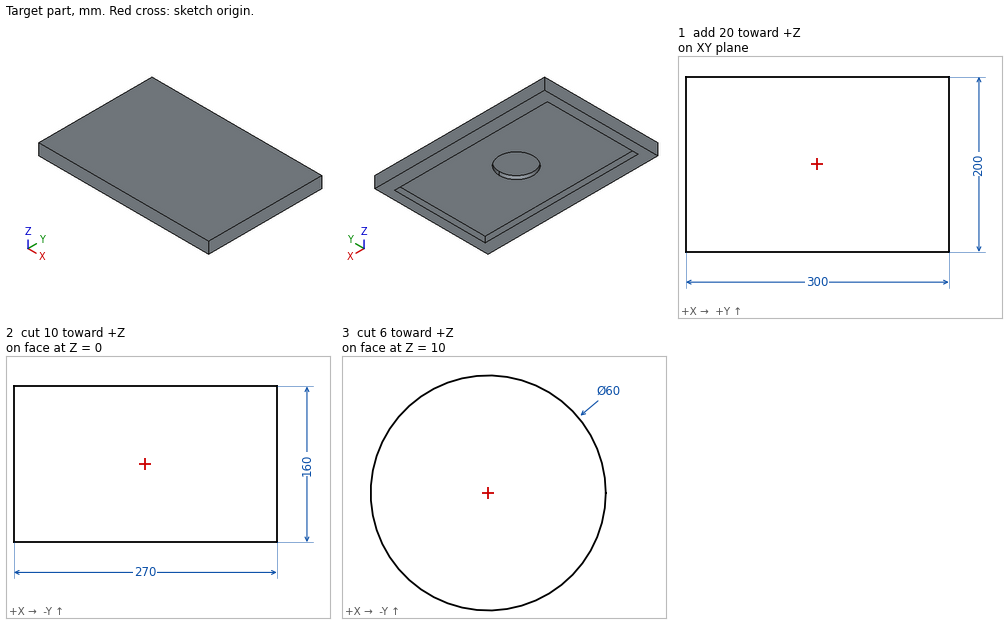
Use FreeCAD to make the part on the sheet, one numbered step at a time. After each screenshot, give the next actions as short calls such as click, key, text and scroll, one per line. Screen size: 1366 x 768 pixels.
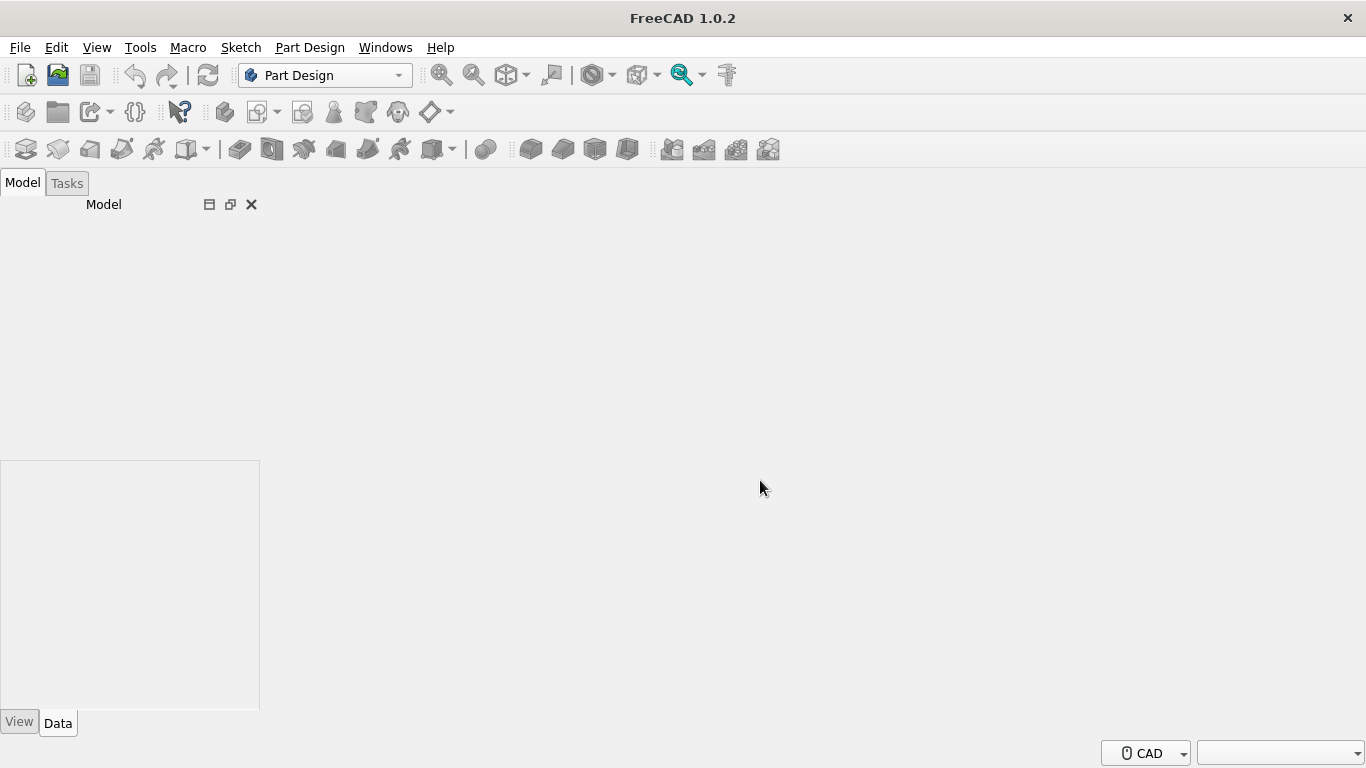
key(ctrl+n)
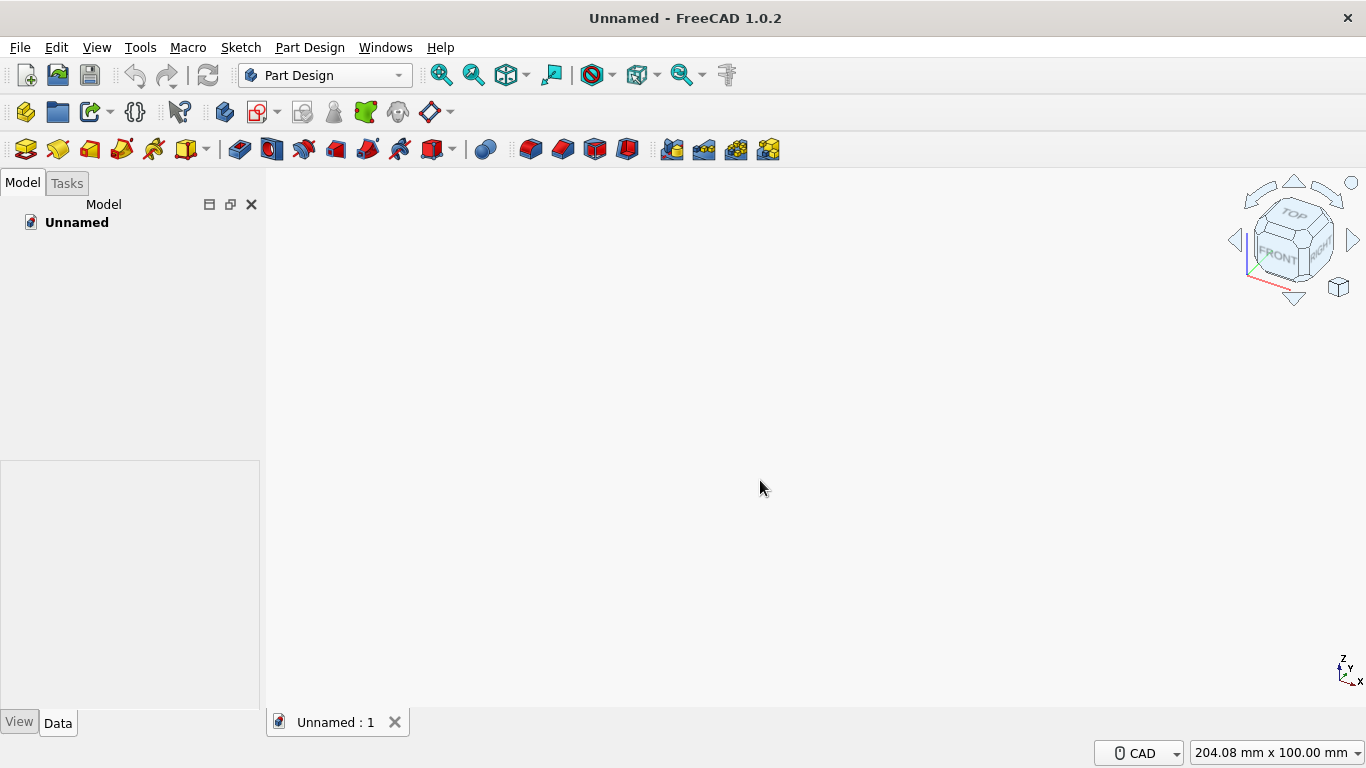
click(258, 112)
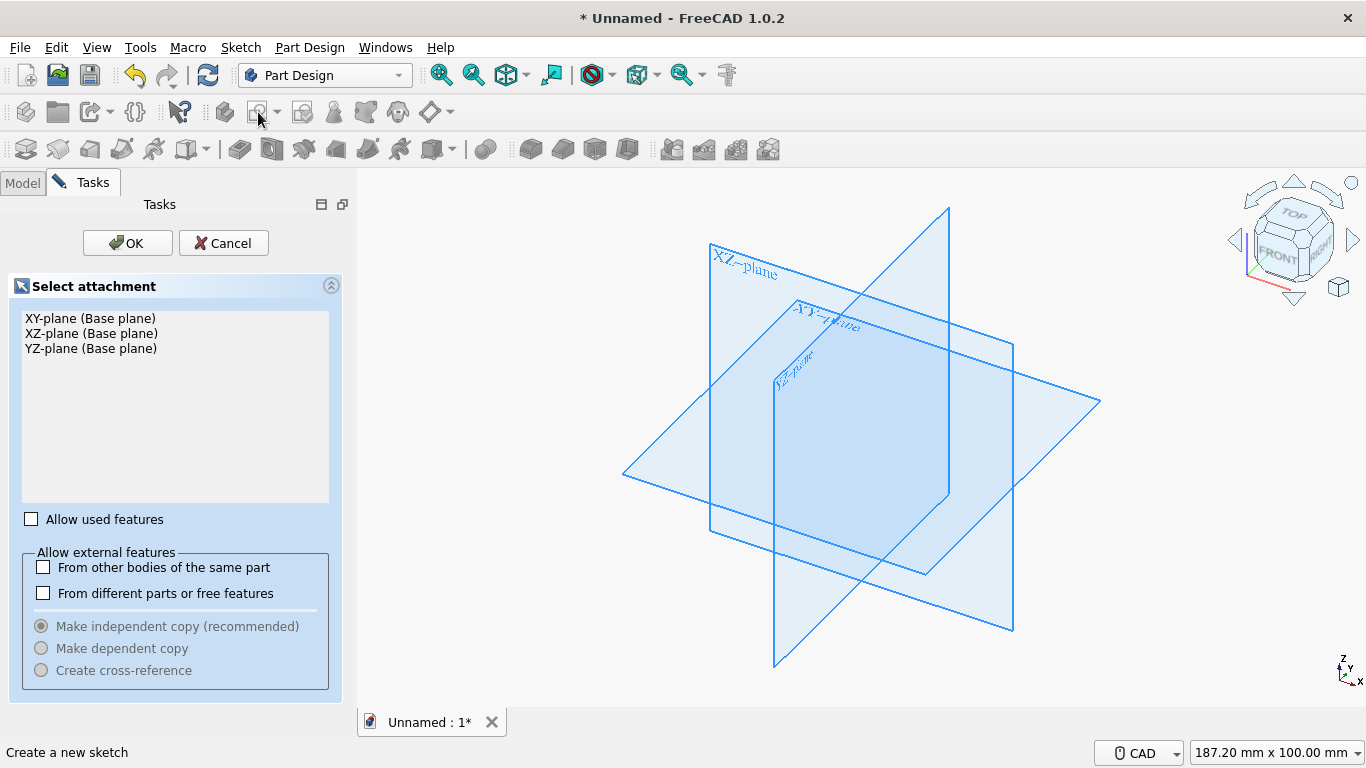
click(82, 318)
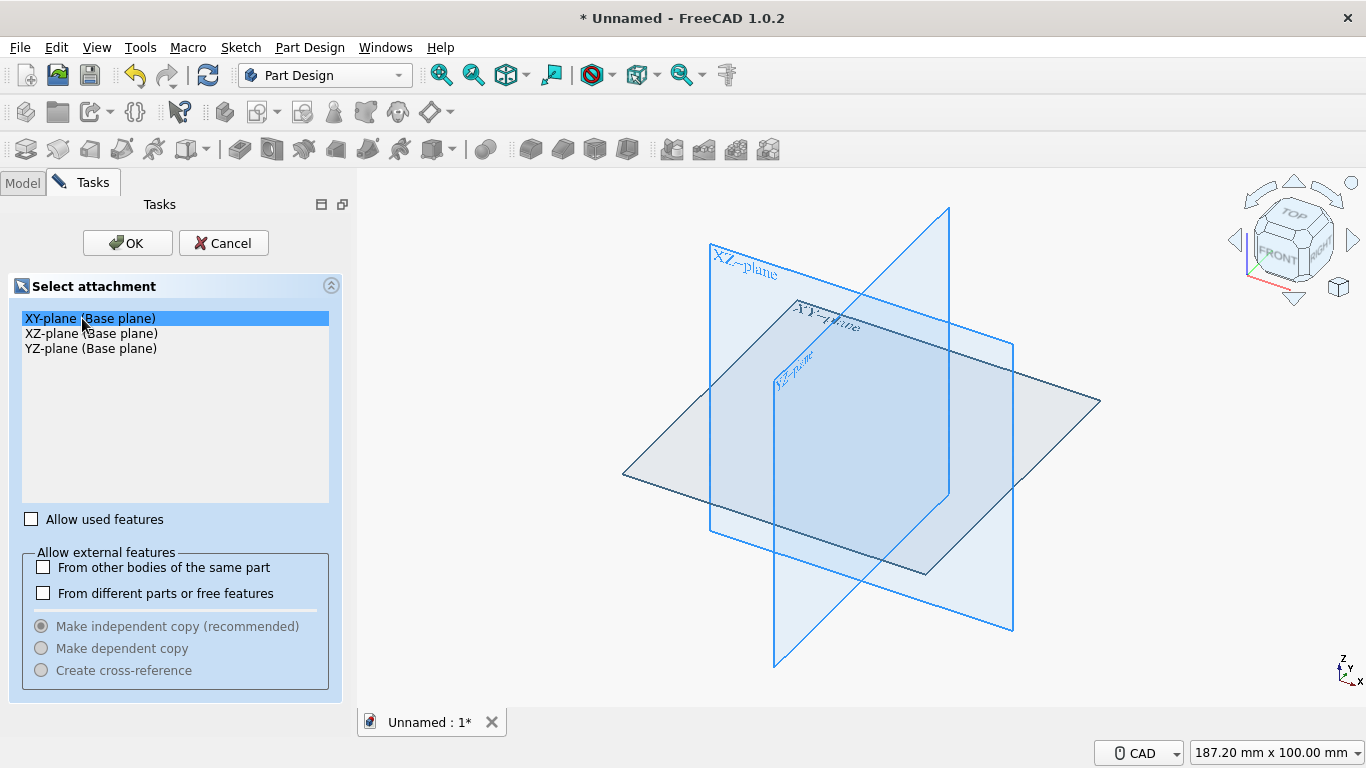
click(128, 243)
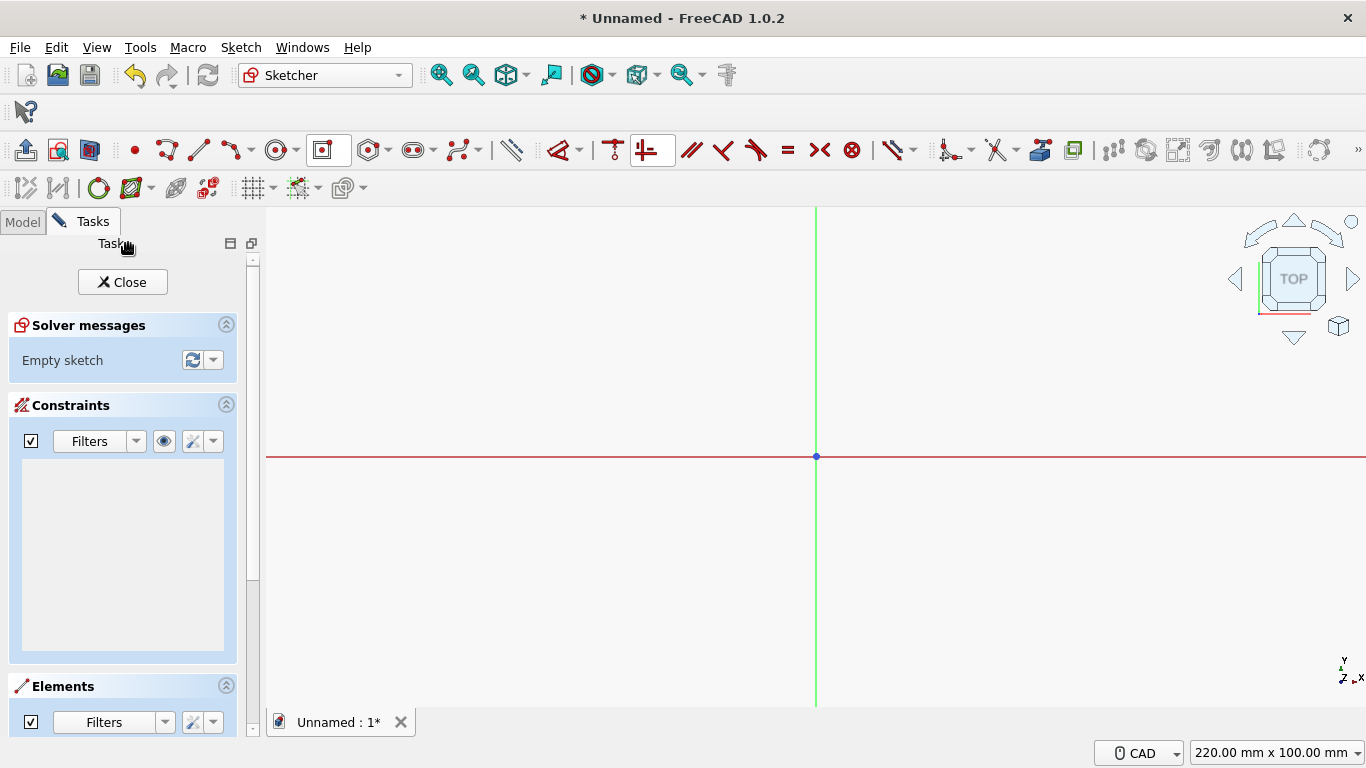
scroll(718, 457, down, 6)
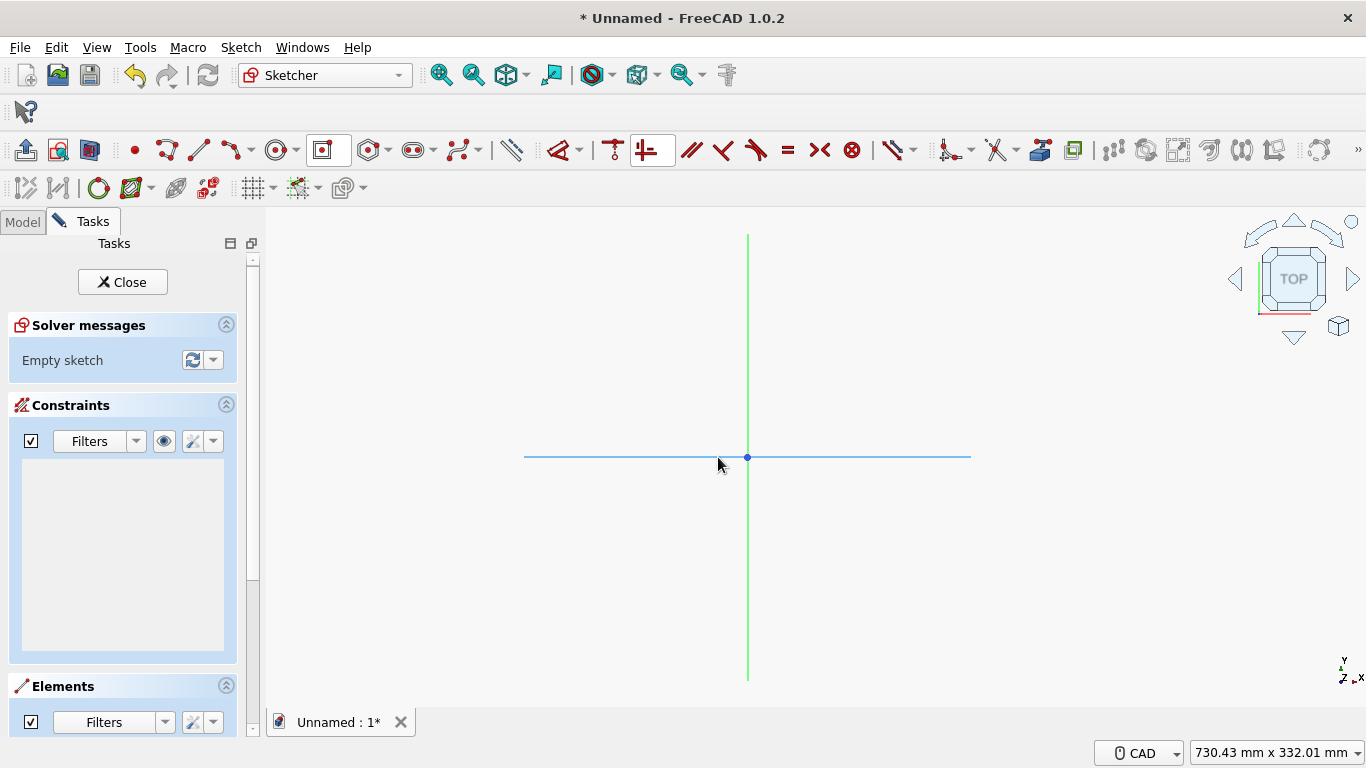
key(g)
key(v)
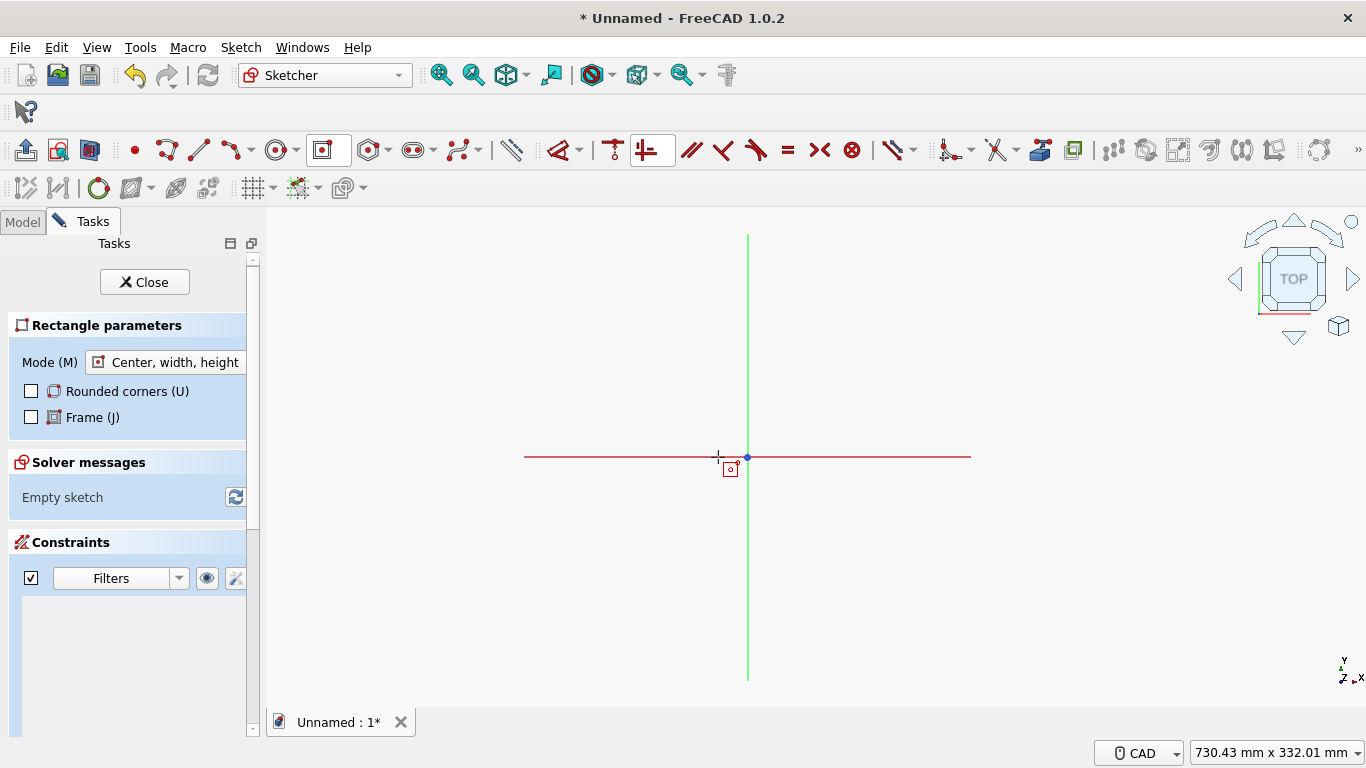
click(748, 457)
click(974, 307)
key(Escape)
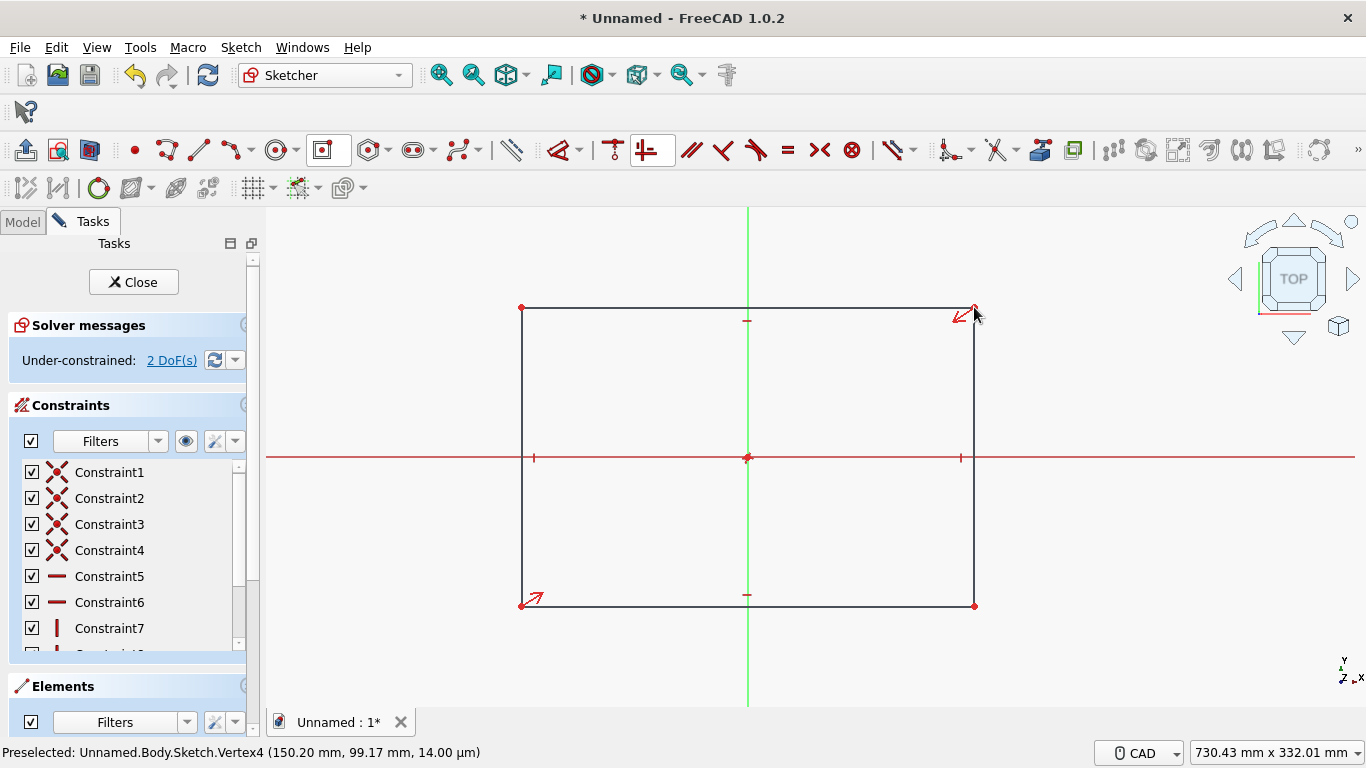
click(657, 607)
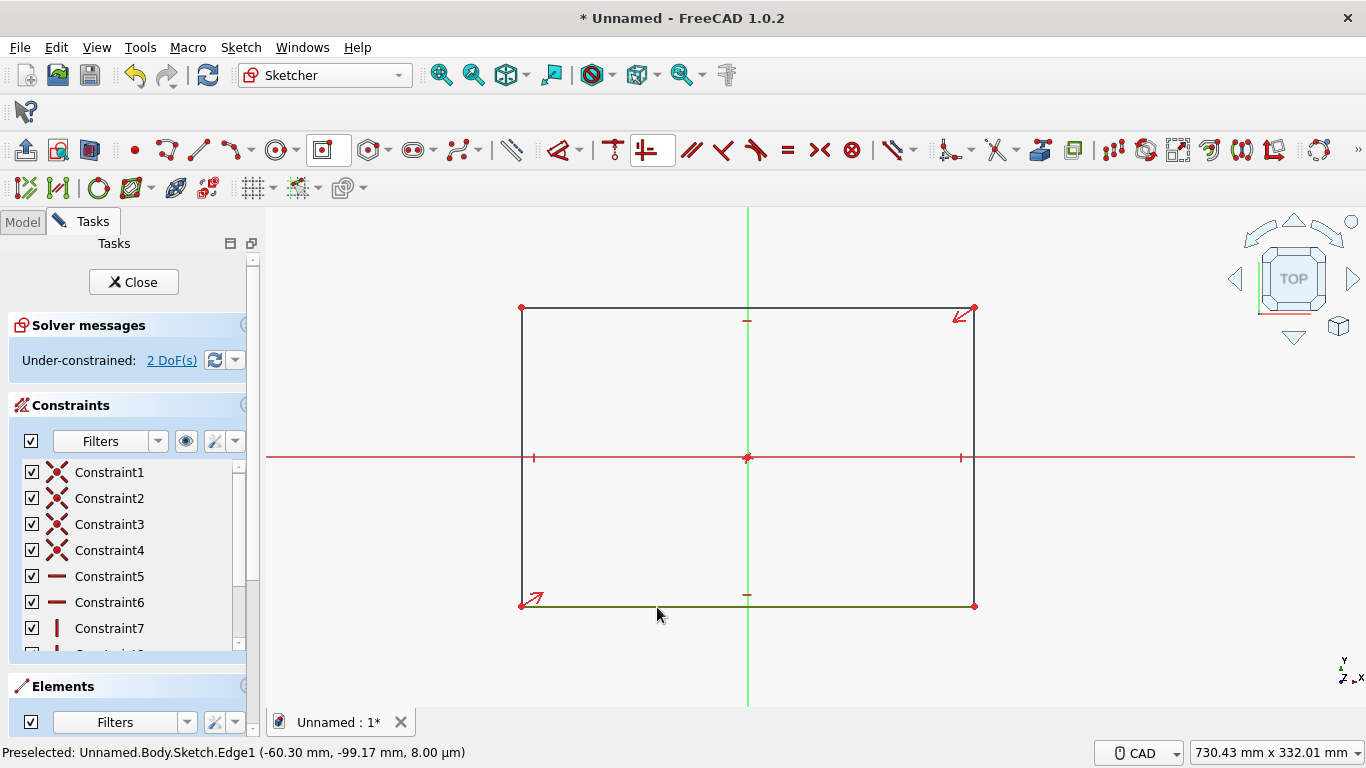
key(l)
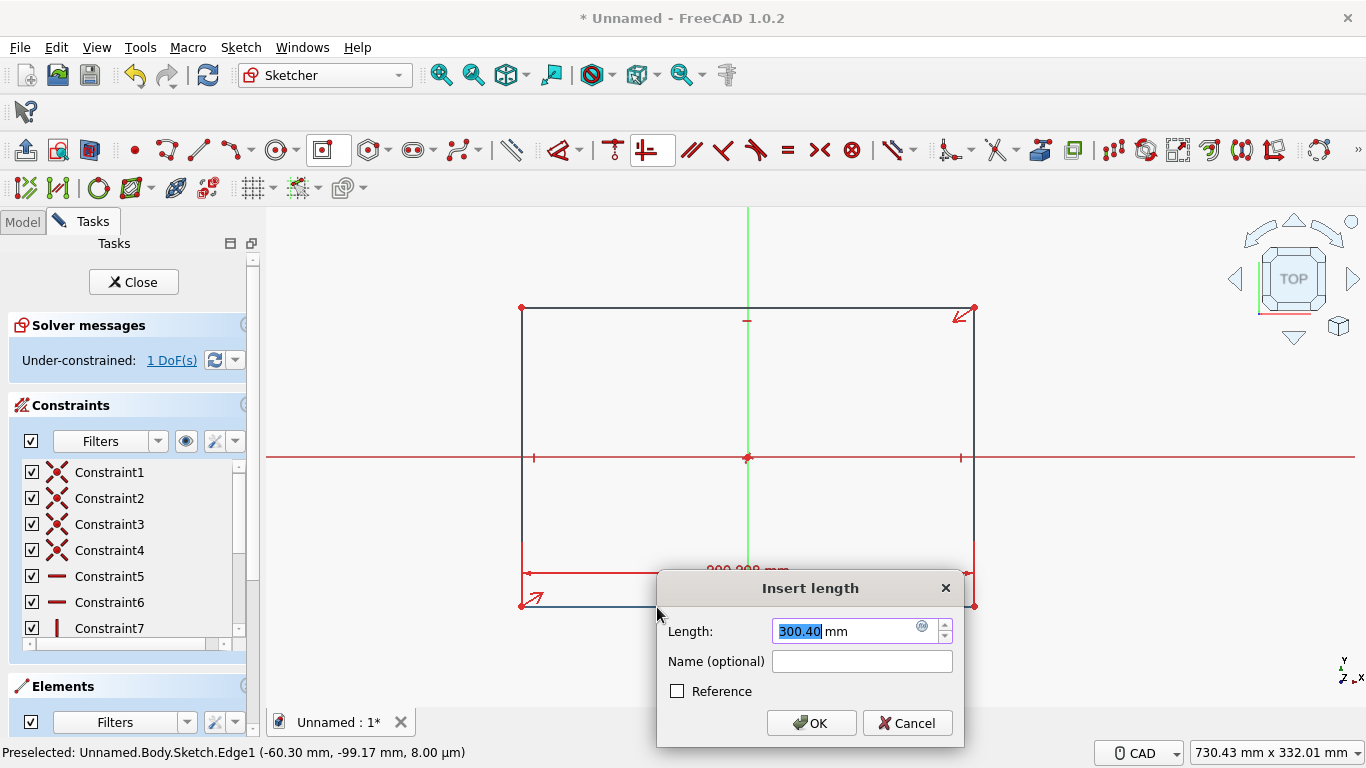
text(300)
key(Return)